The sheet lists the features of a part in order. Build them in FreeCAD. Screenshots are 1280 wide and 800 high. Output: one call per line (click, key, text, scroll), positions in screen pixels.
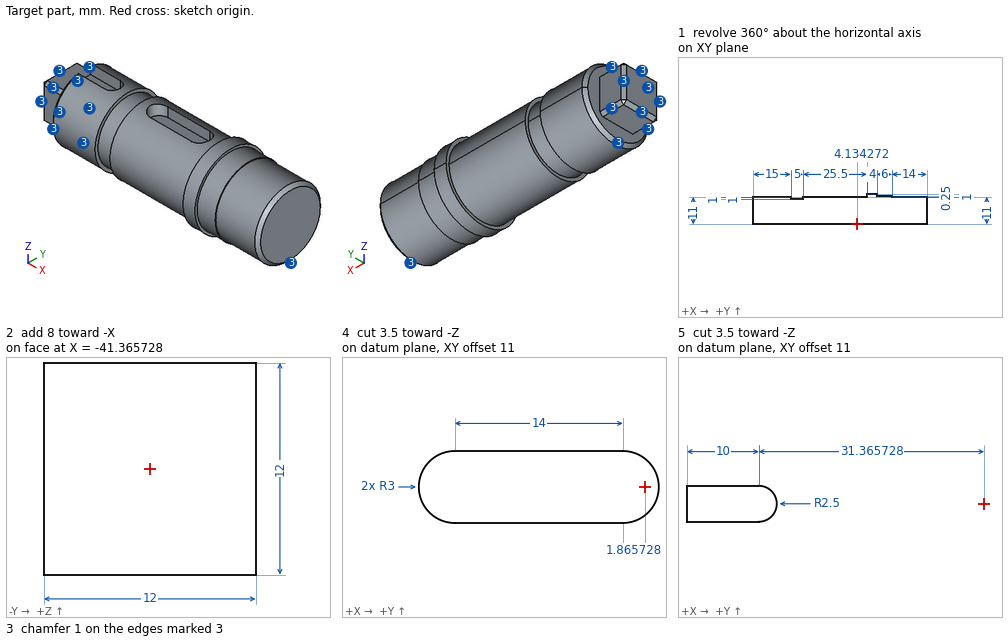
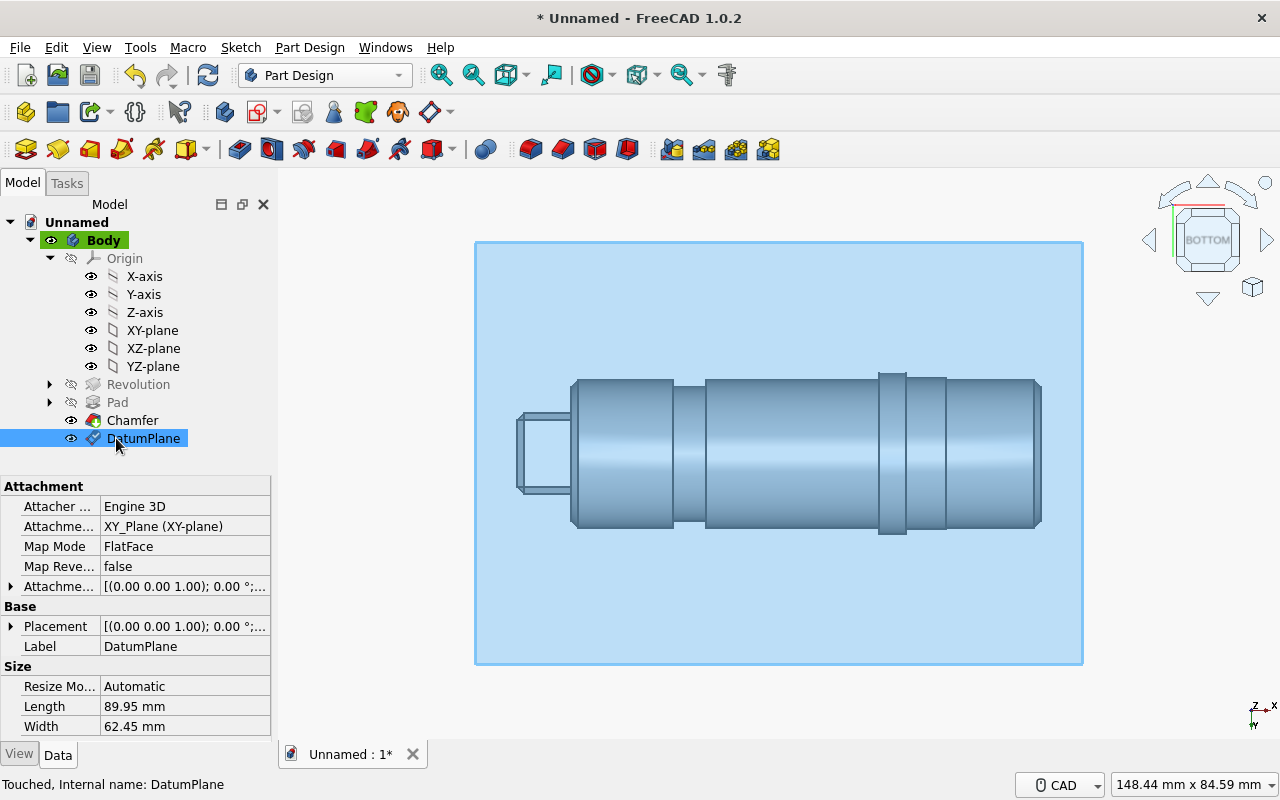
click(258, 112)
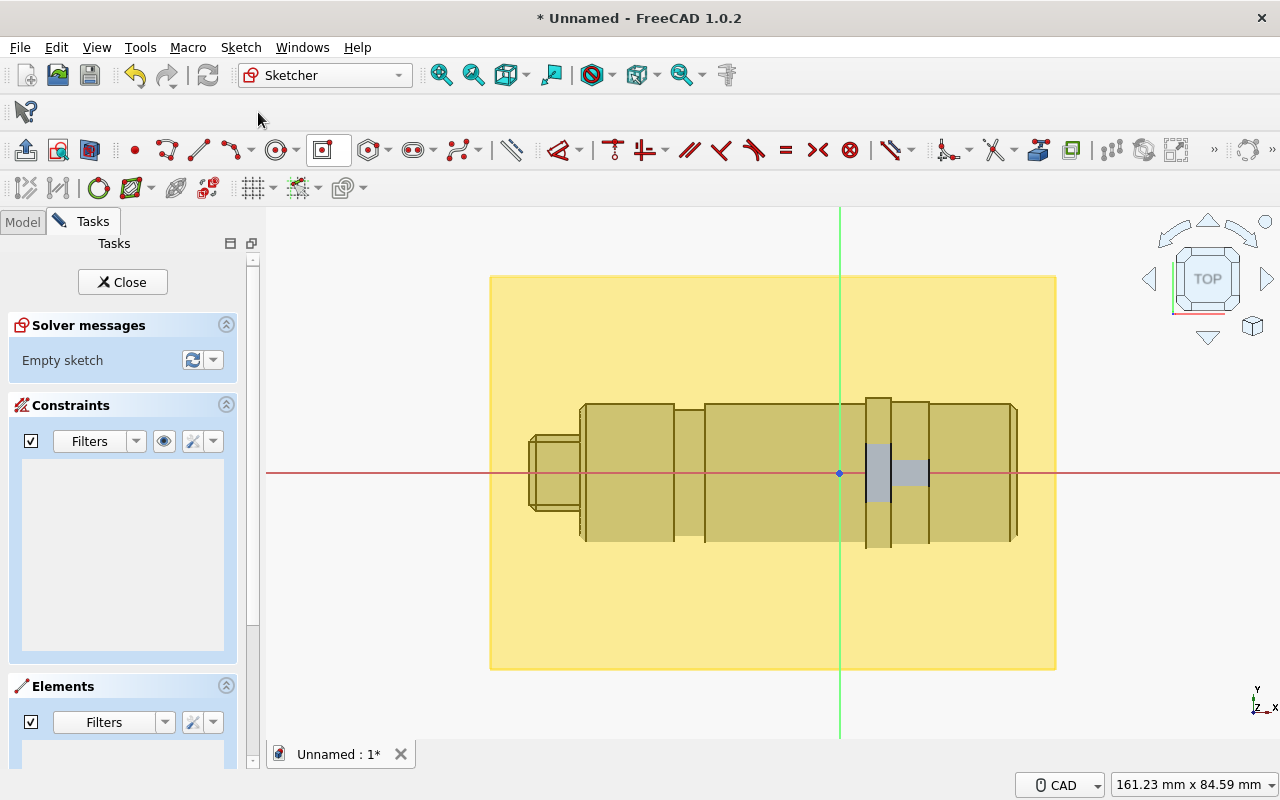
key(q)
key(s)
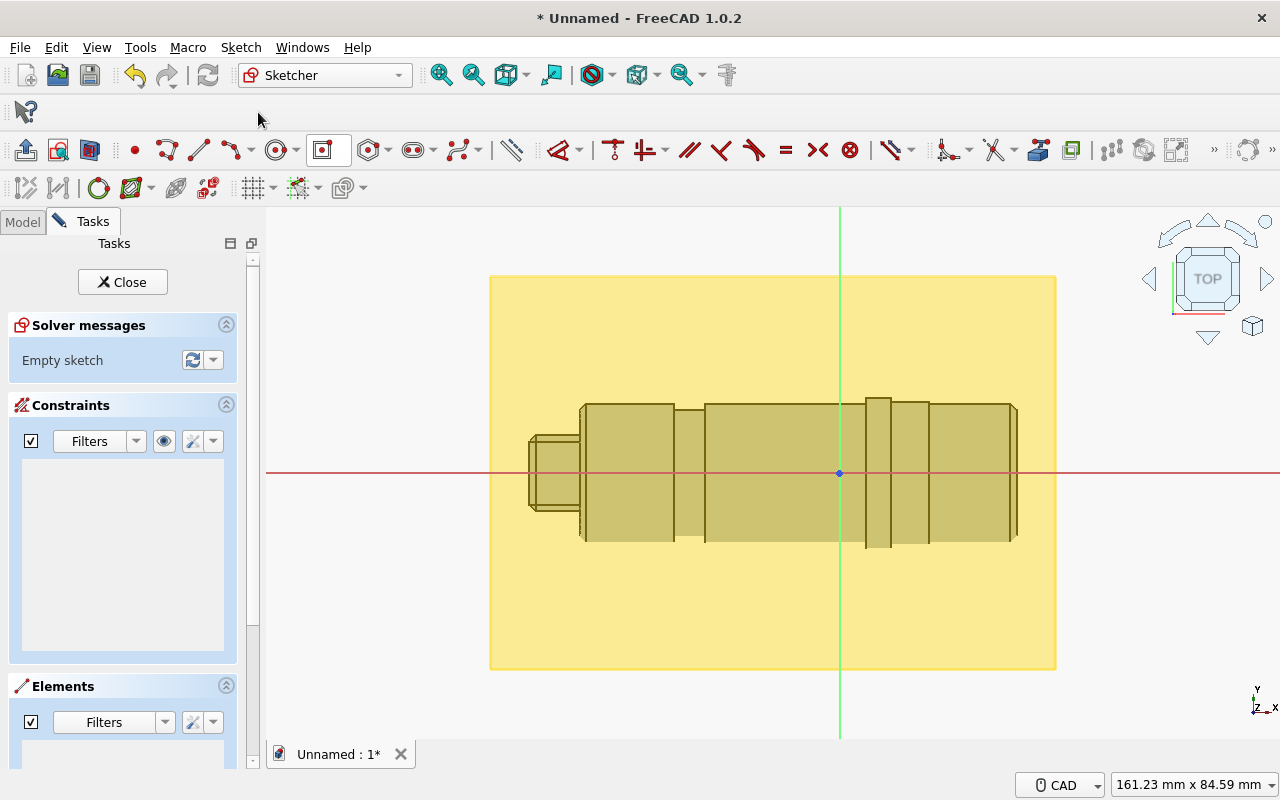
scroll(804, 473, up, 8)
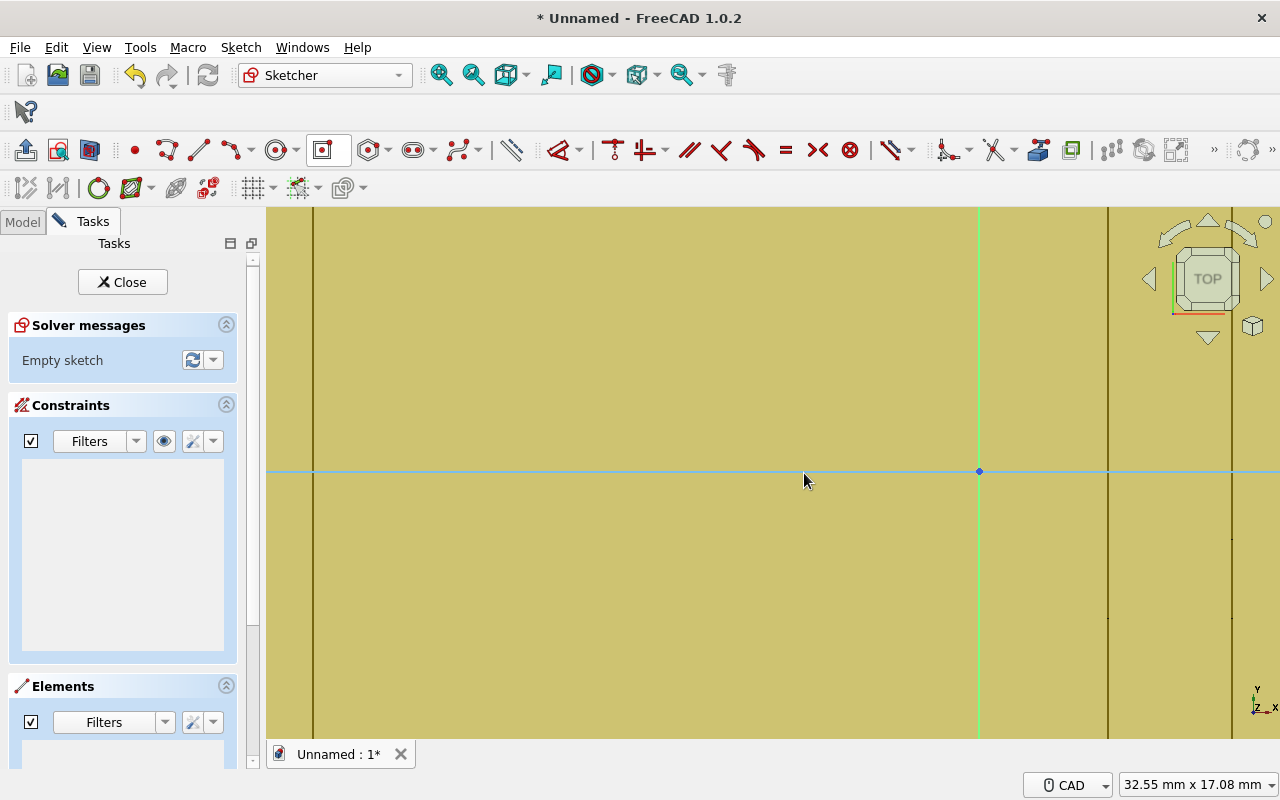
click(414, 150)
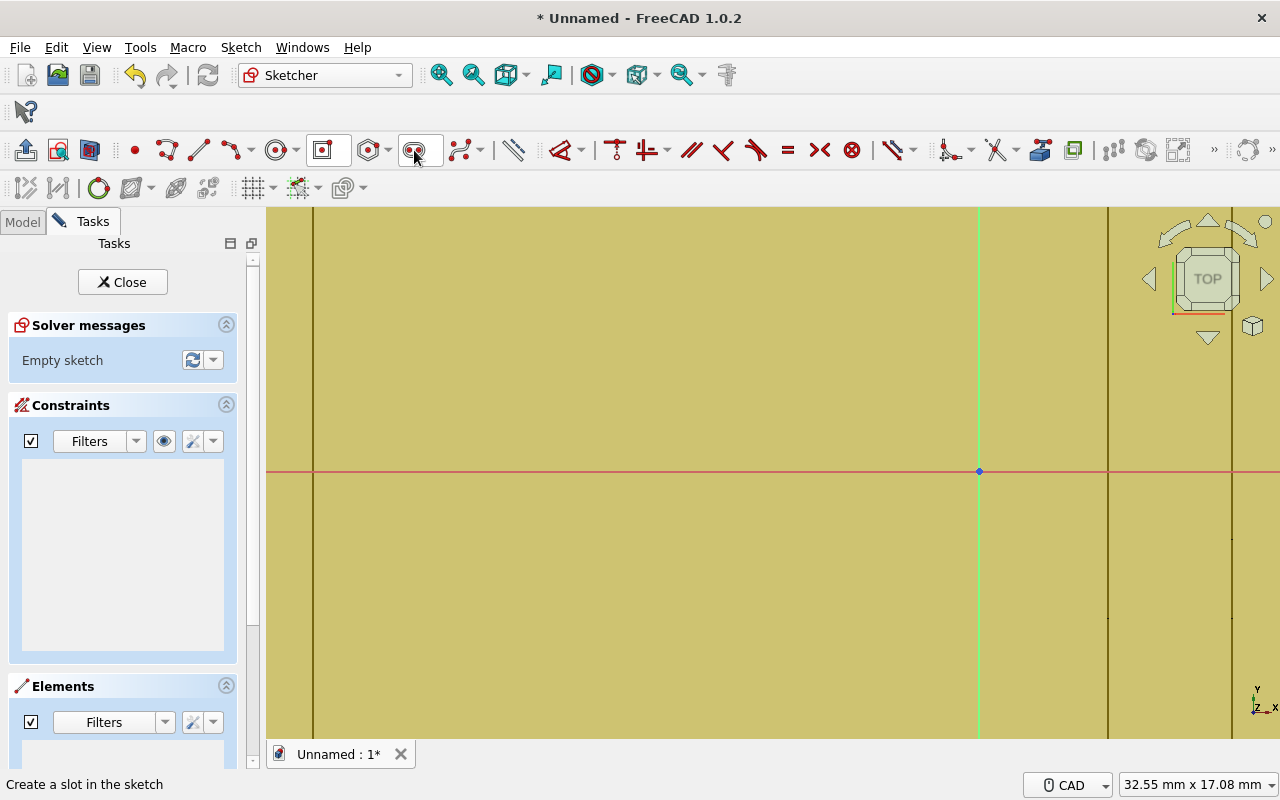
click(485, 472)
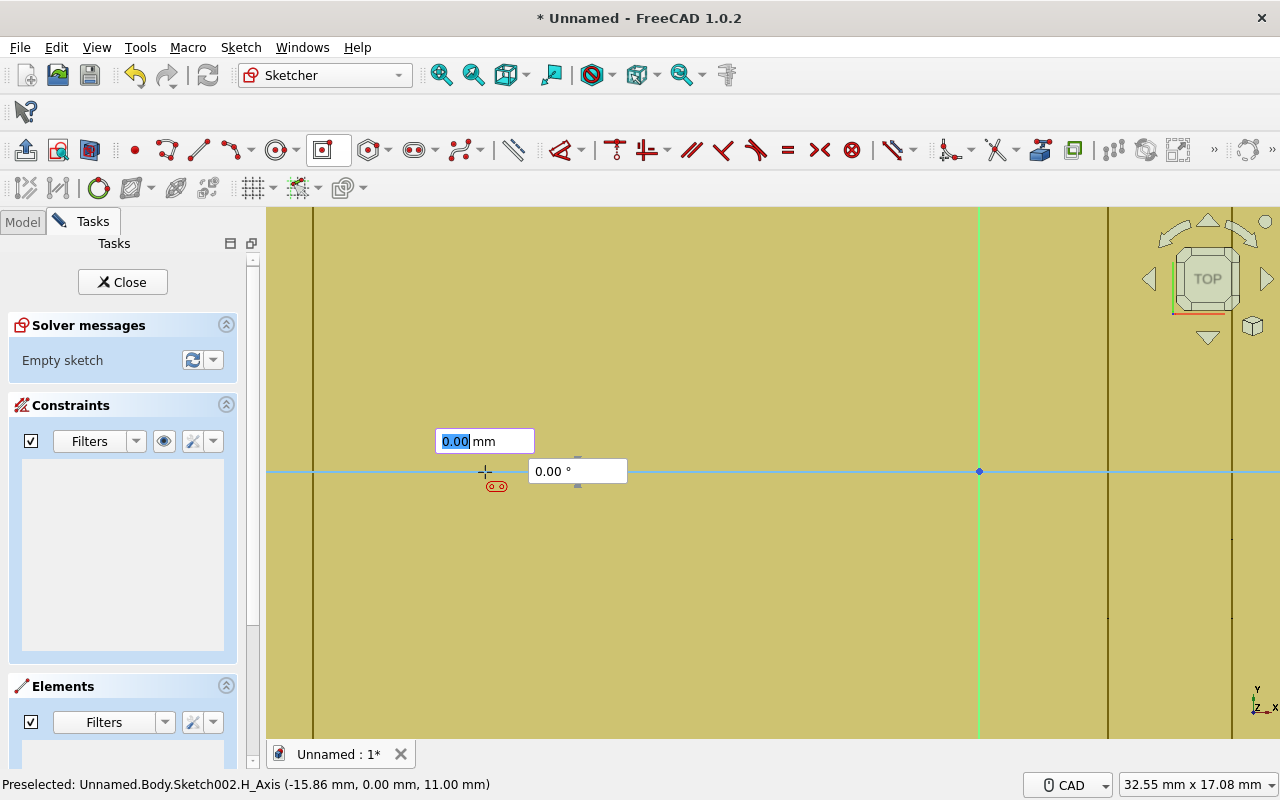
click(921, 463)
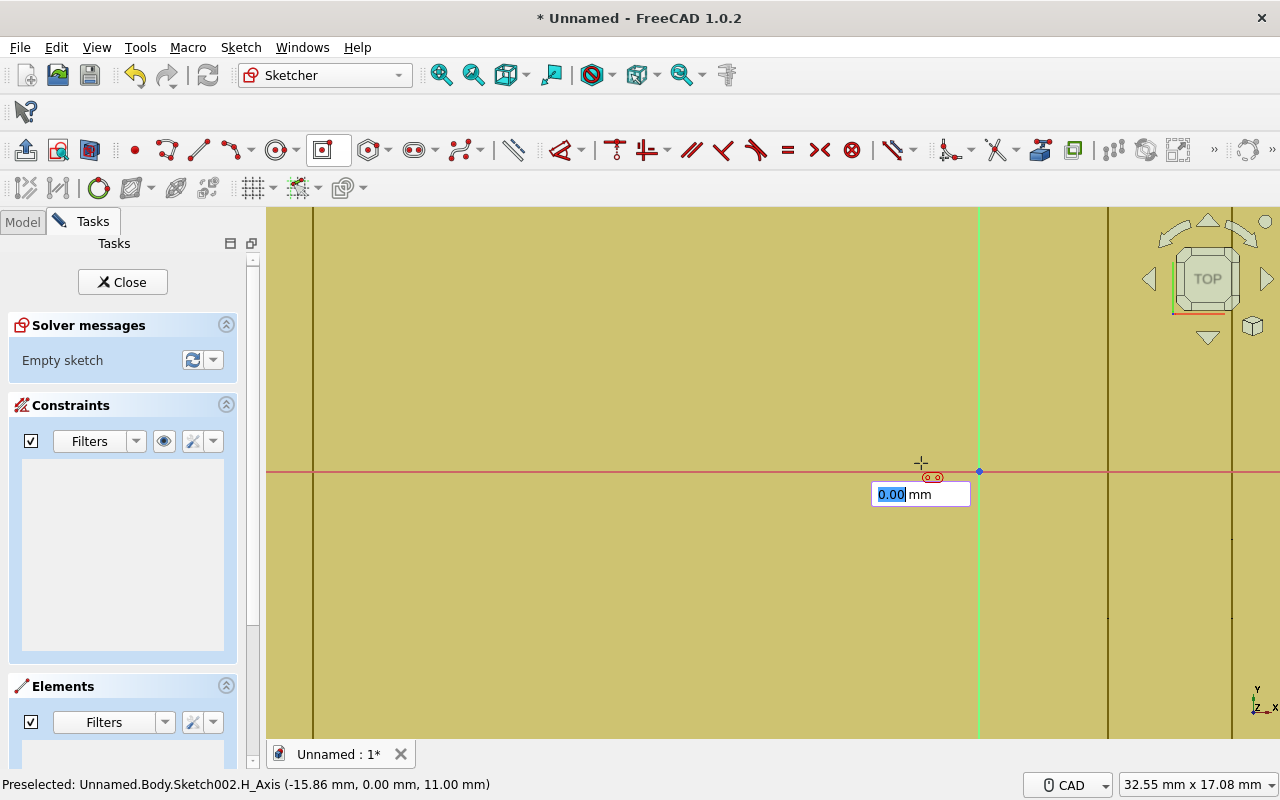
click(703, 378)
key(Escape)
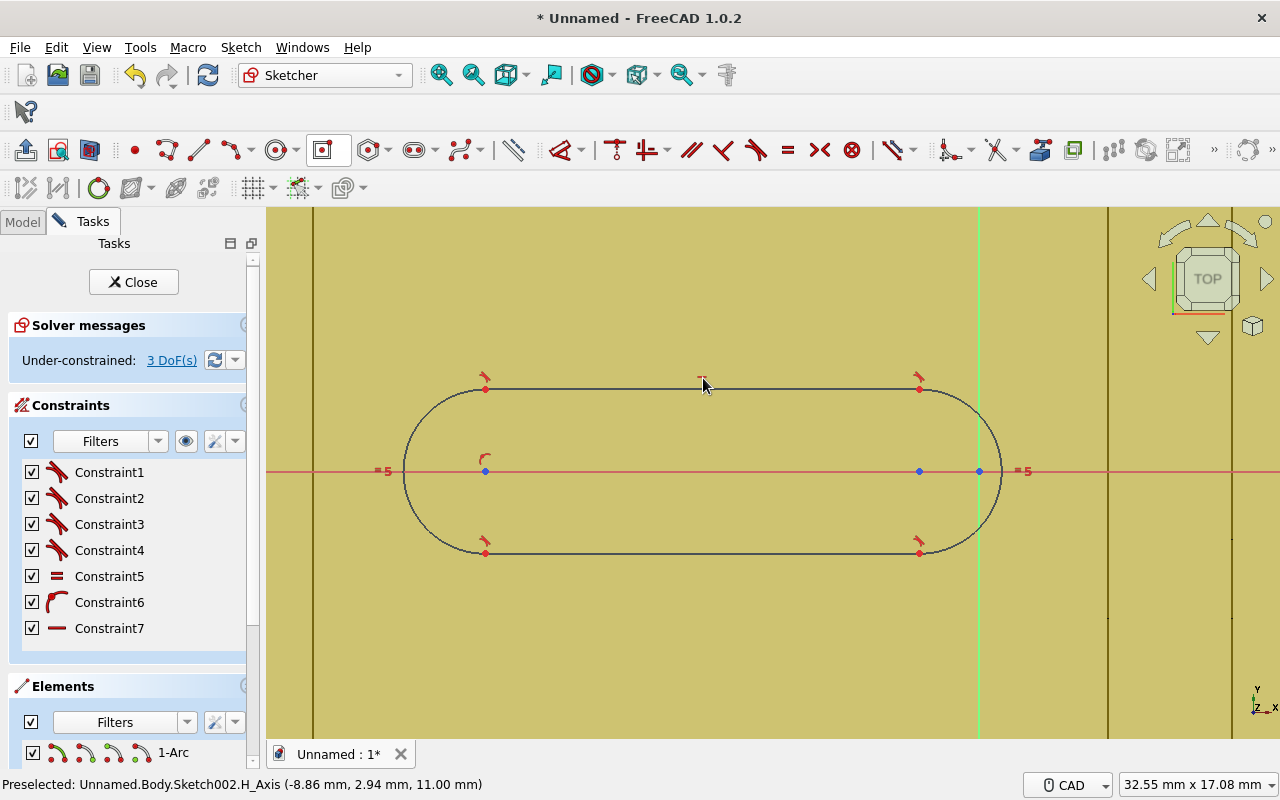
click(560, 150)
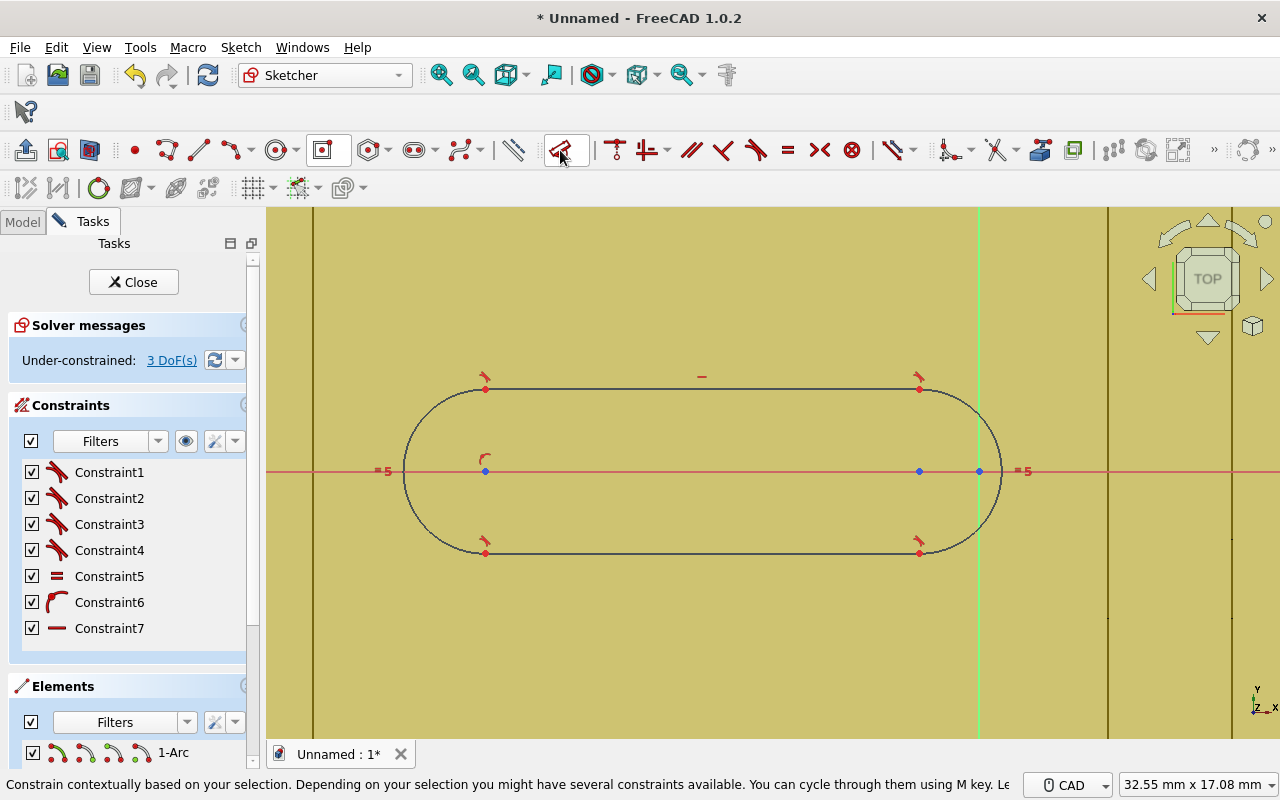
click(419, 423)
click(393, 404)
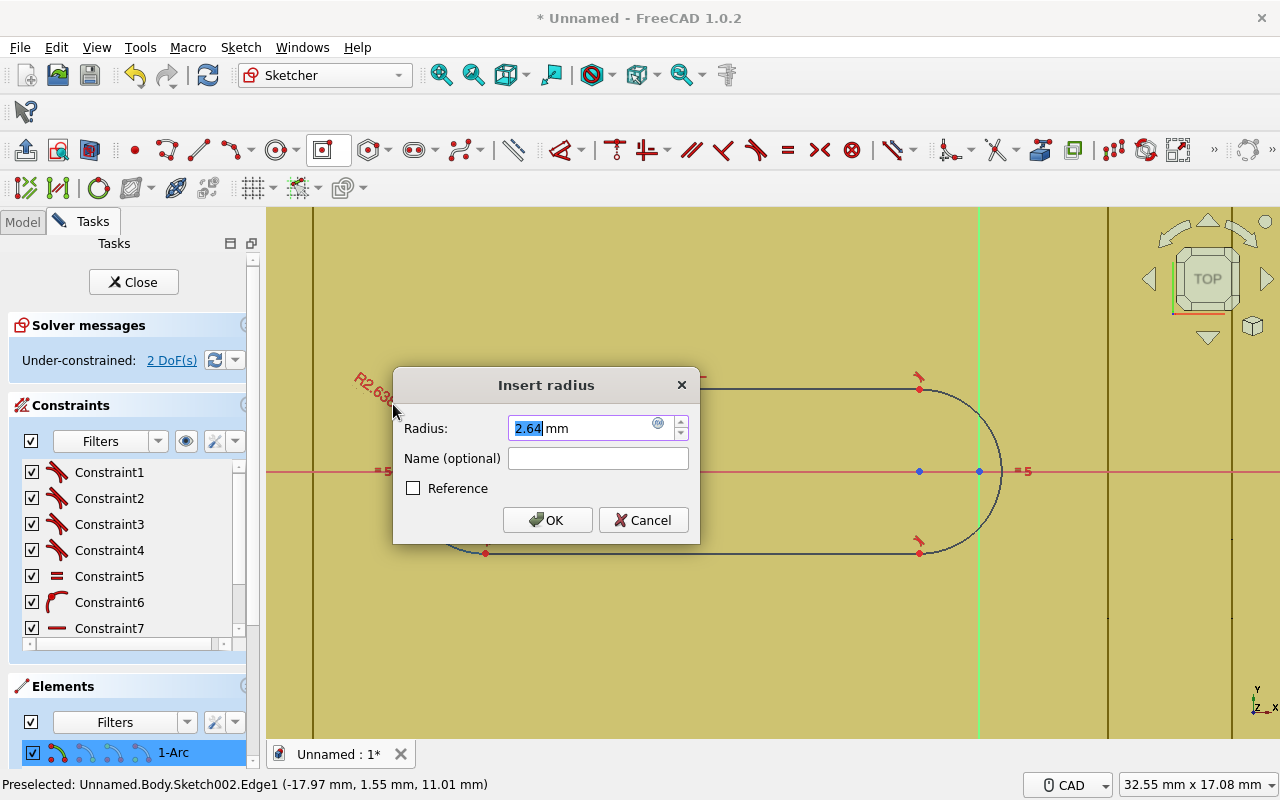
text(3)
key(Return)